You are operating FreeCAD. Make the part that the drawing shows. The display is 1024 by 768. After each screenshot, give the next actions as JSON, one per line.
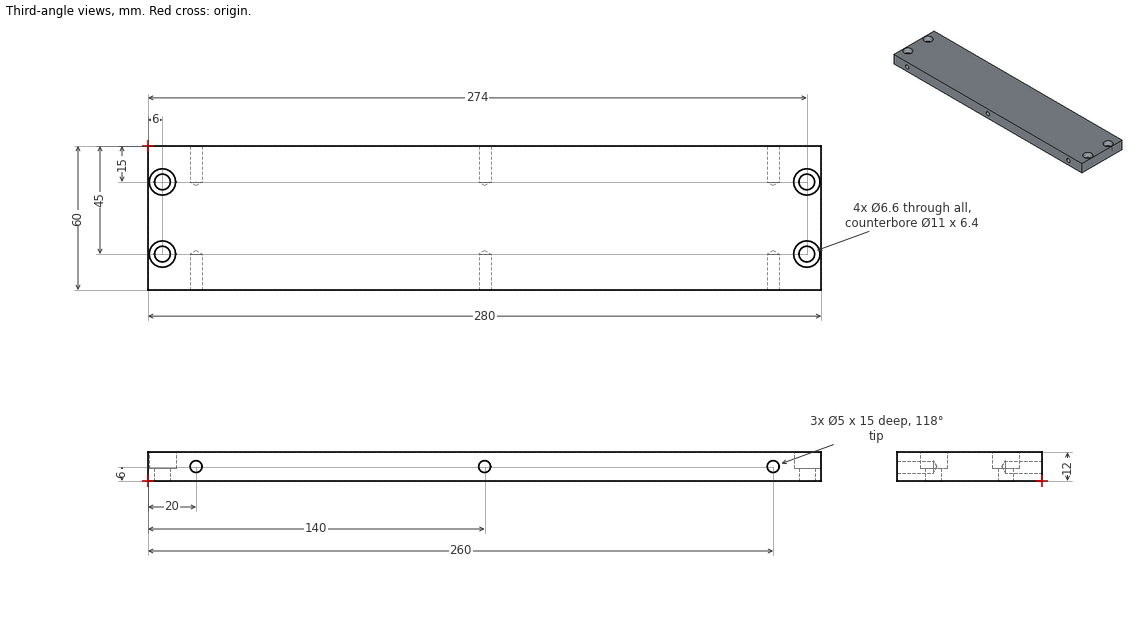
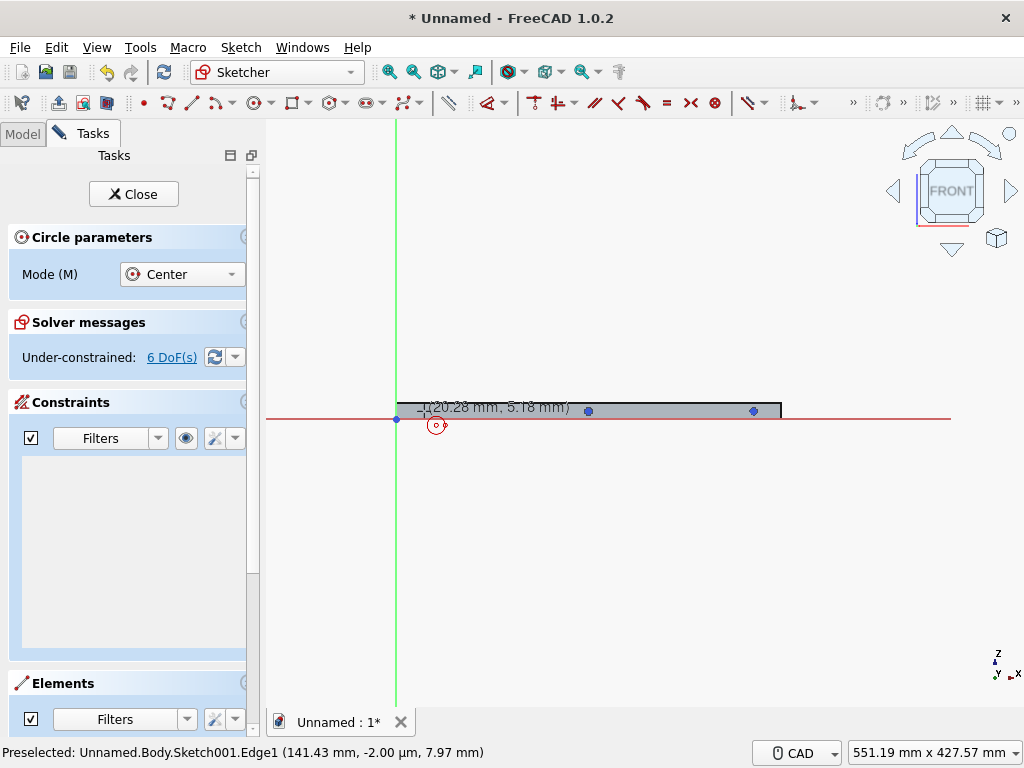
{"action": "scroll", "coordinate": [424, 411], "scroll_direction": "up", "scroll_amount": 4}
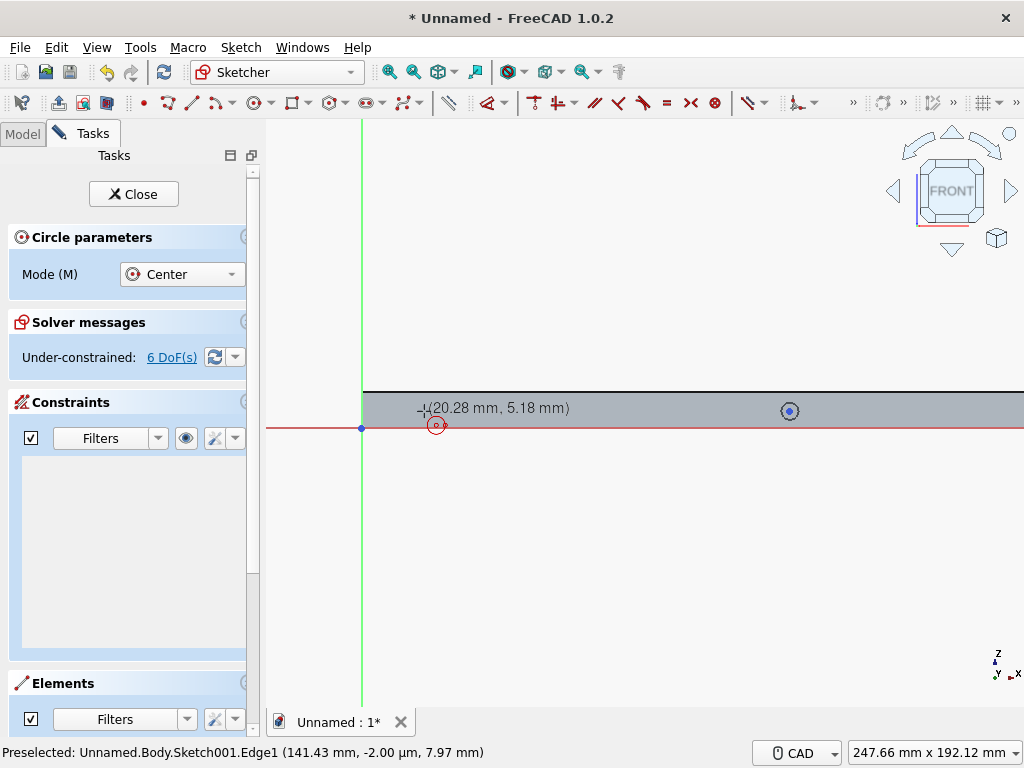
{"action": "left_click", "coordinate": [423, 410]}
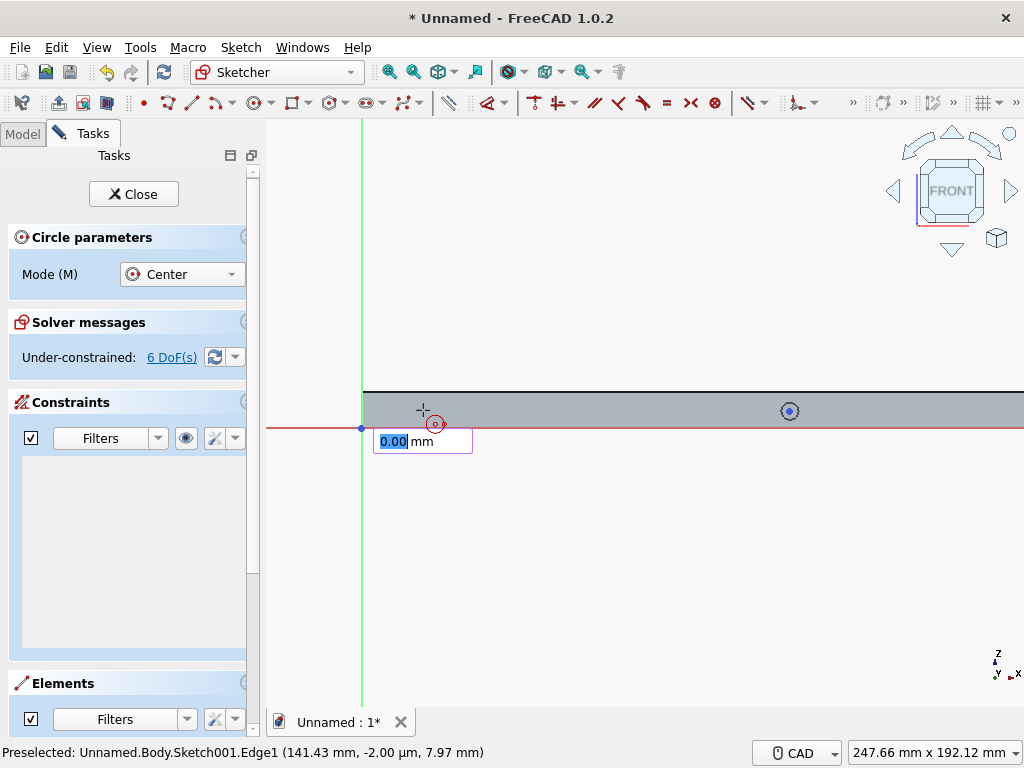
{"action": "scroll", "coordinate": [428, 405], "scroll_direction": "up", "scroll_amount": 4}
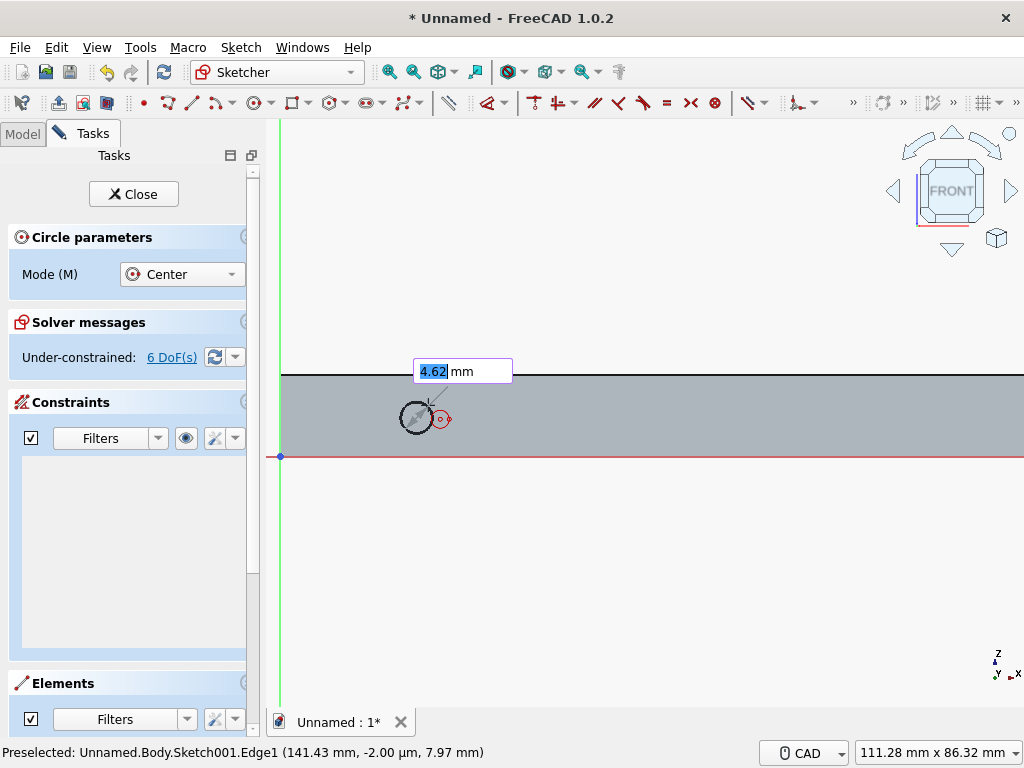
{"action": "left_click", "coordinate": [428, 404]}
{"action": "key", "text": "Escape"}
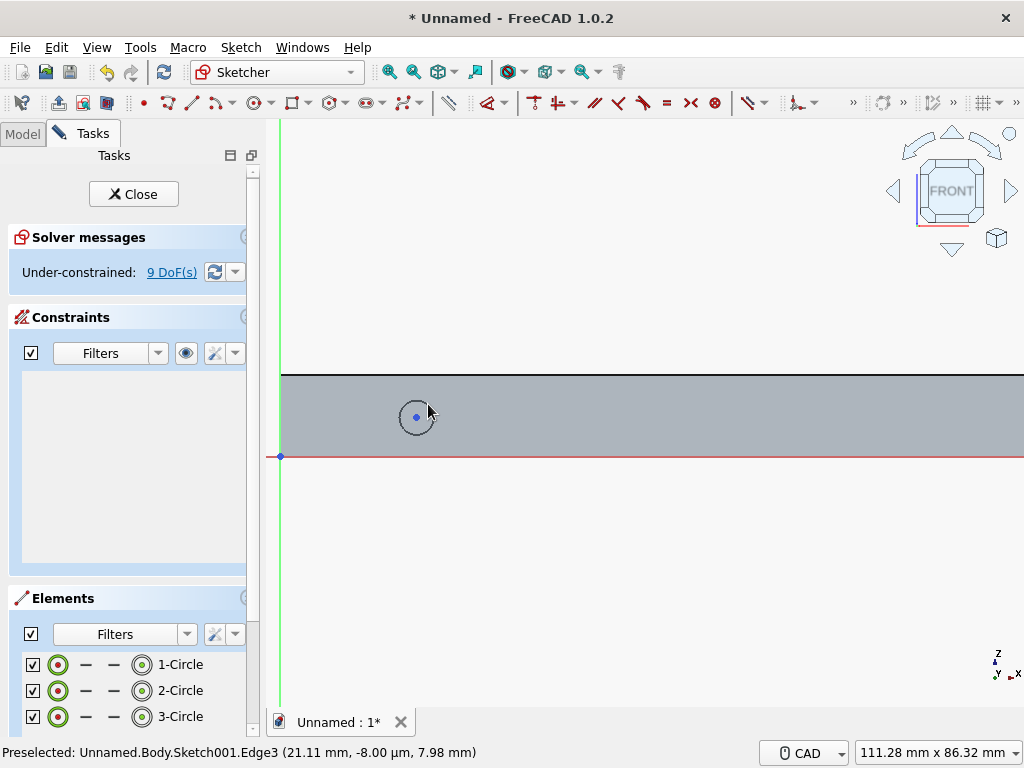
{"action": "scroll", "coordinate": [425, 409], "scroll_direction": "down", "scroll_amount": 8}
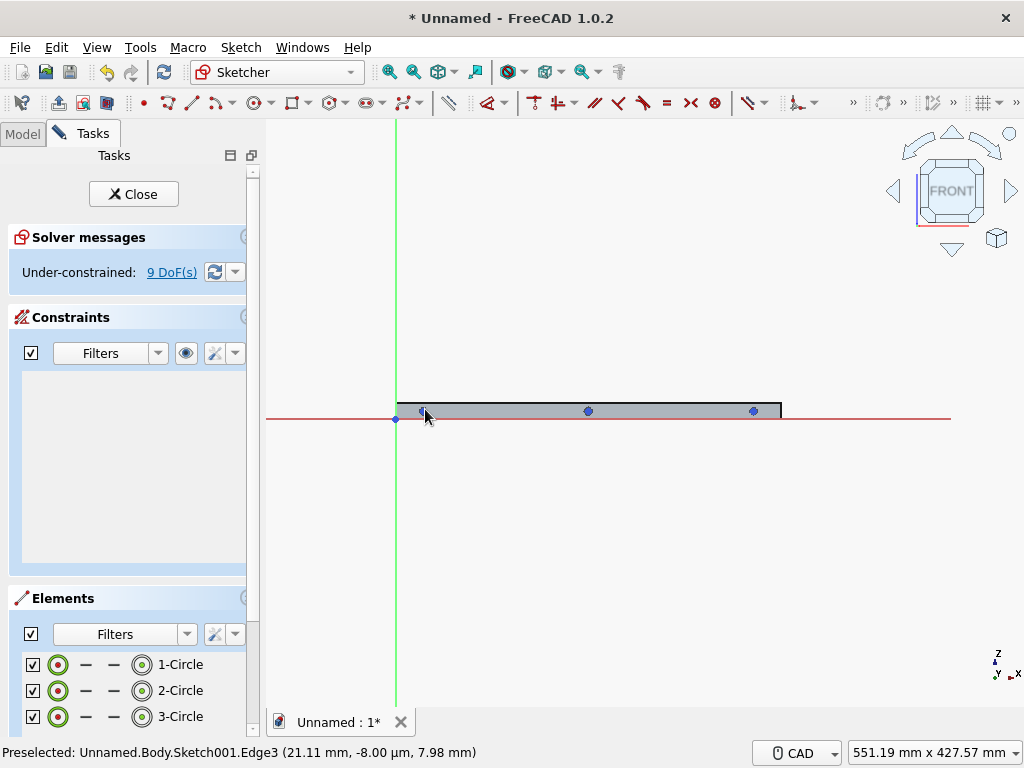
{"action": "scroll", "coordinate": [756, 409], "scroll_direction": "up", "scroll_amount": 8}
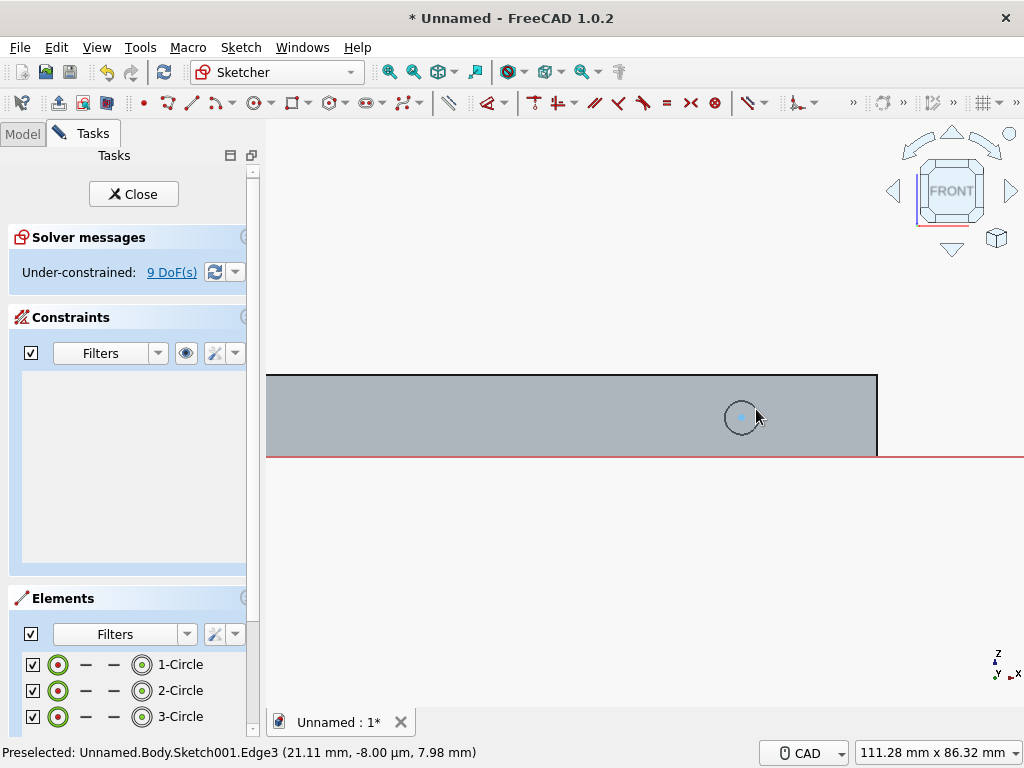
{"action": "left_click", "coordinate": [754, 406]}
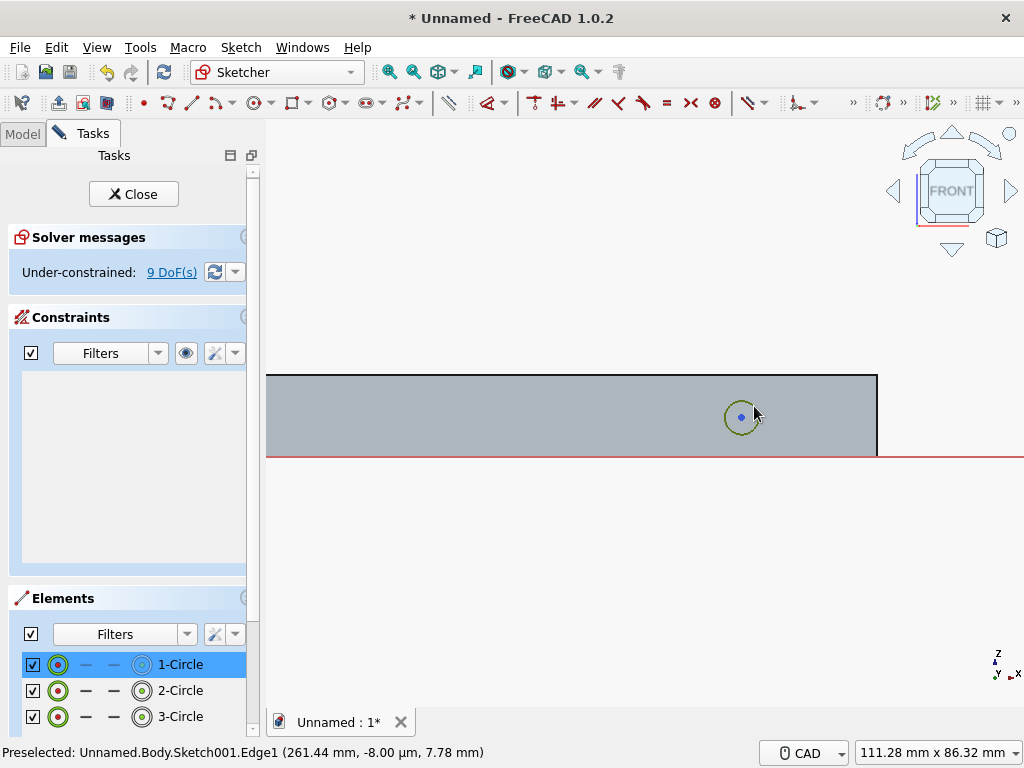
{"action": "scroll", "coordinate": [757, 409], "scroll_direction": "down", "scroll_amount": 8}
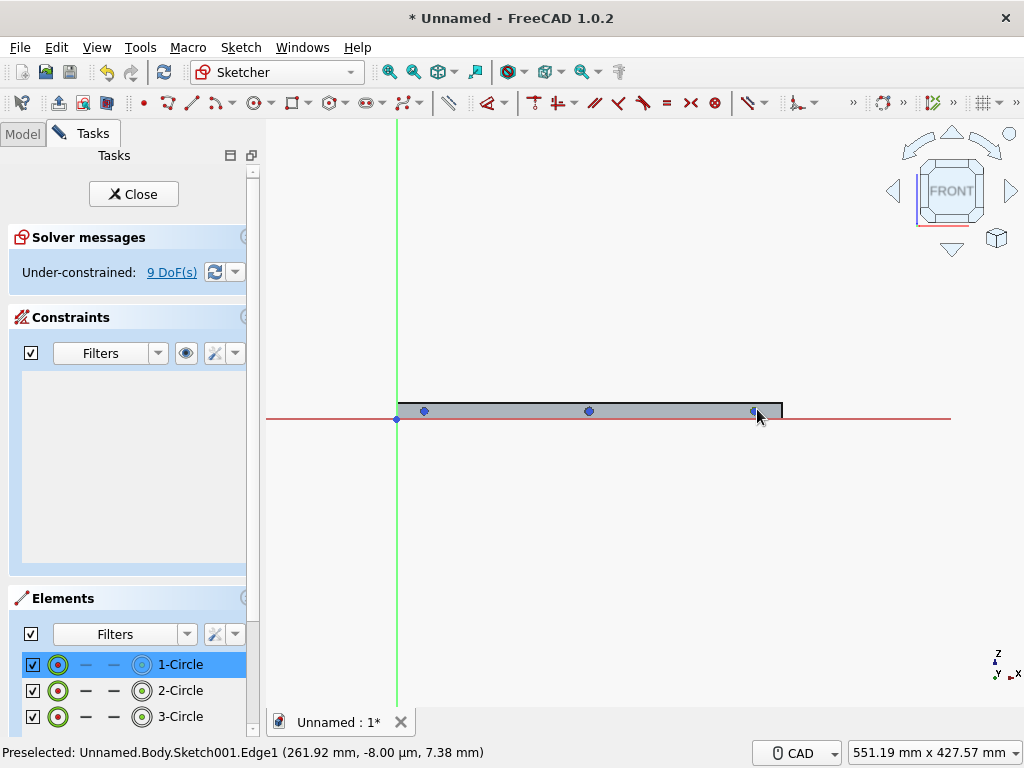
{"action": "scroll", "coordinate": [592, 409], "scroll_direction": "up", "scroll_amount": 7}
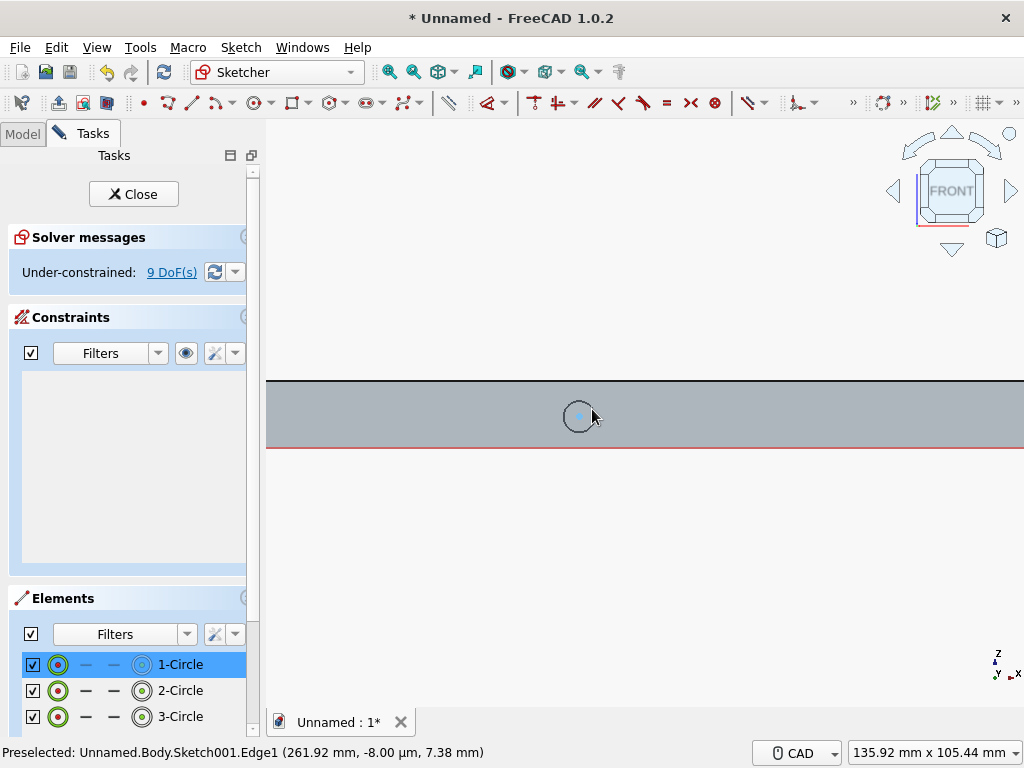
{"action": "left_click", "coordinate": [590, 406]}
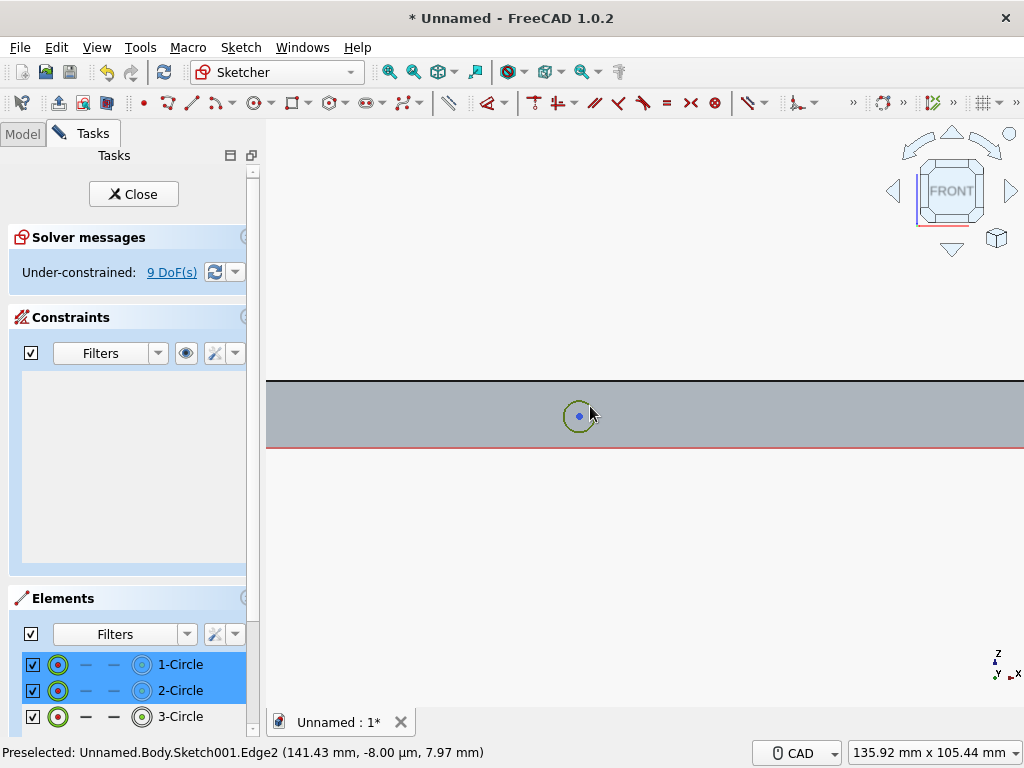
{"action": "scroll", "coordinate": [591, 409], "scroll_direction": "down", "scroll_amount": 7}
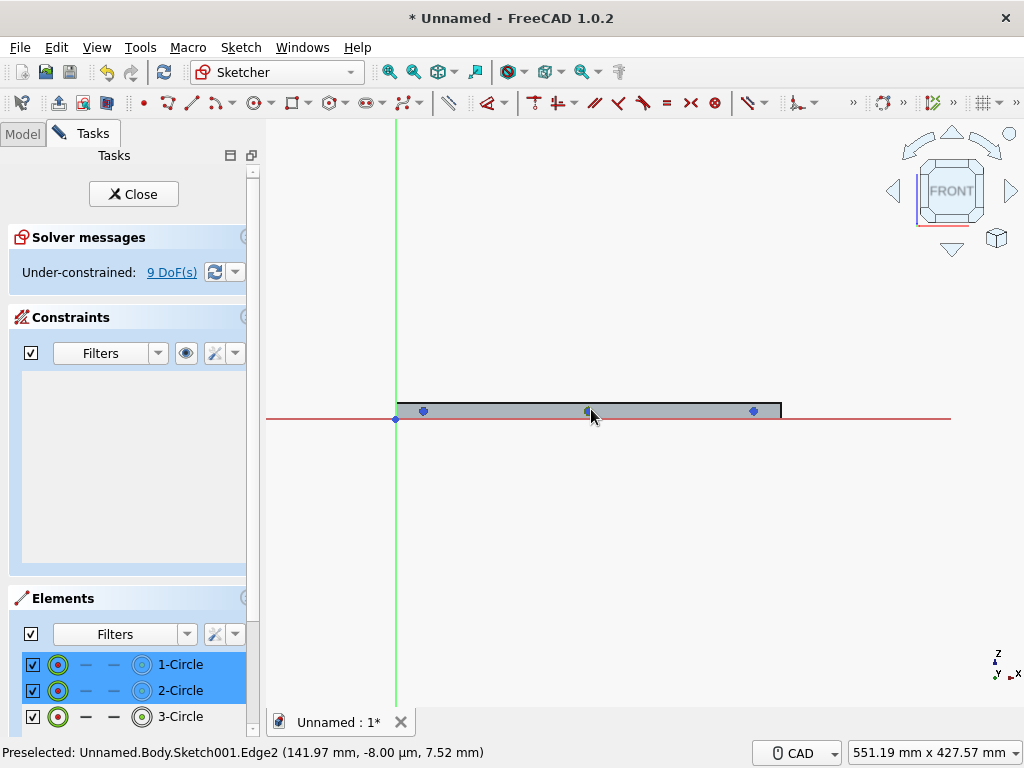
{"action": "scroll", "coordinate": [426, 409], "scroll_direction": "up", "scroll_amount": 7}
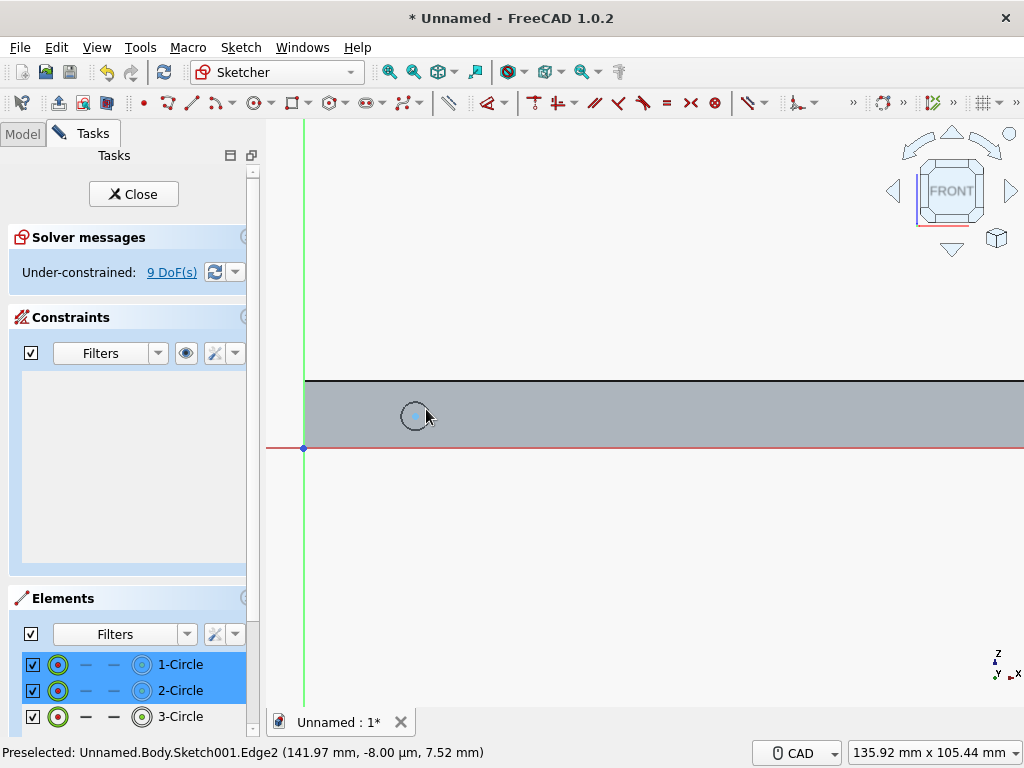
{"action": "left_click", "coordinate": [425, 406]}